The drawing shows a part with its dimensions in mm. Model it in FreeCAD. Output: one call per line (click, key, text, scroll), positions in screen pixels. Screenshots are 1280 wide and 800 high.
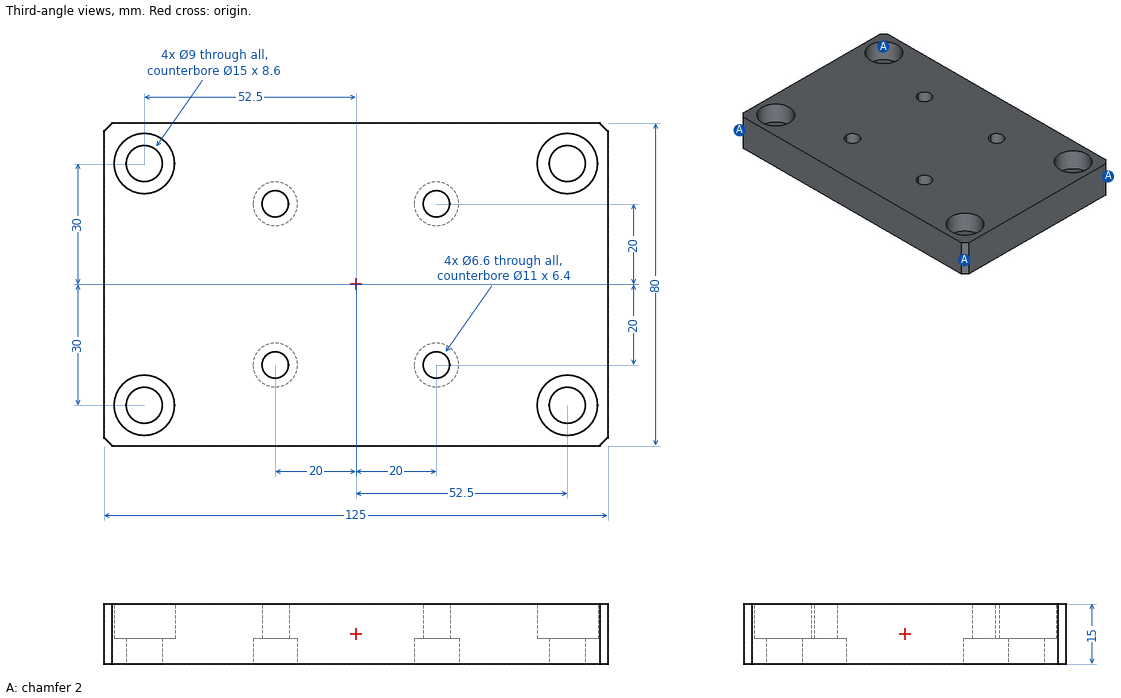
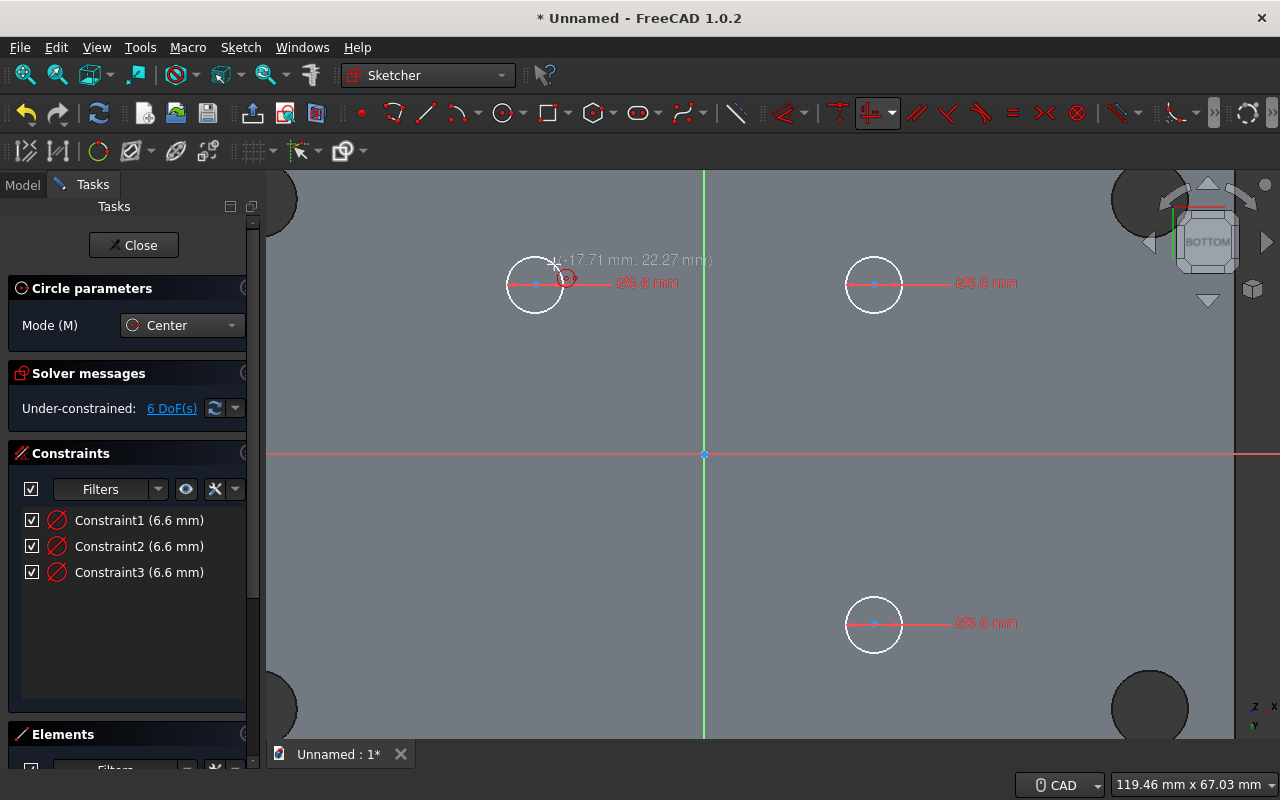
click(535, 624)
move(554, 604)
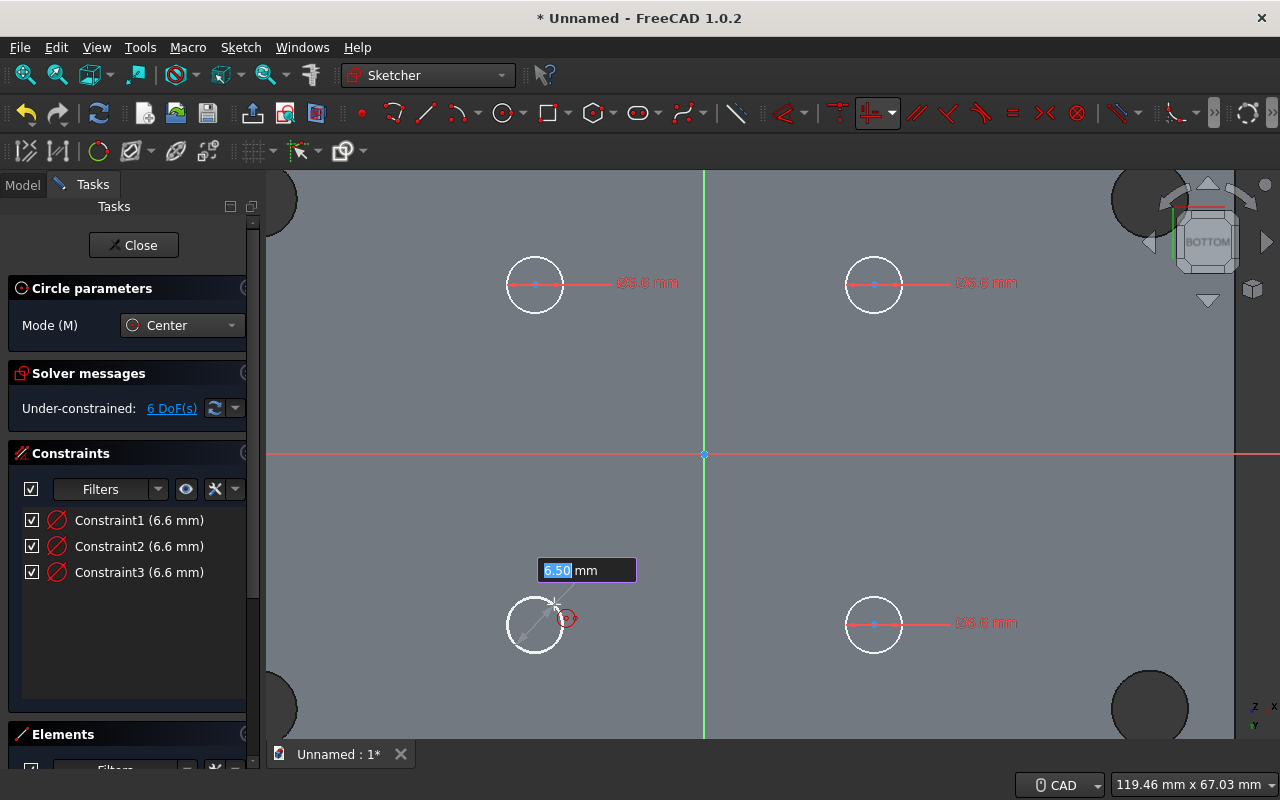
text(6.6)
key(Return)
key(Escape)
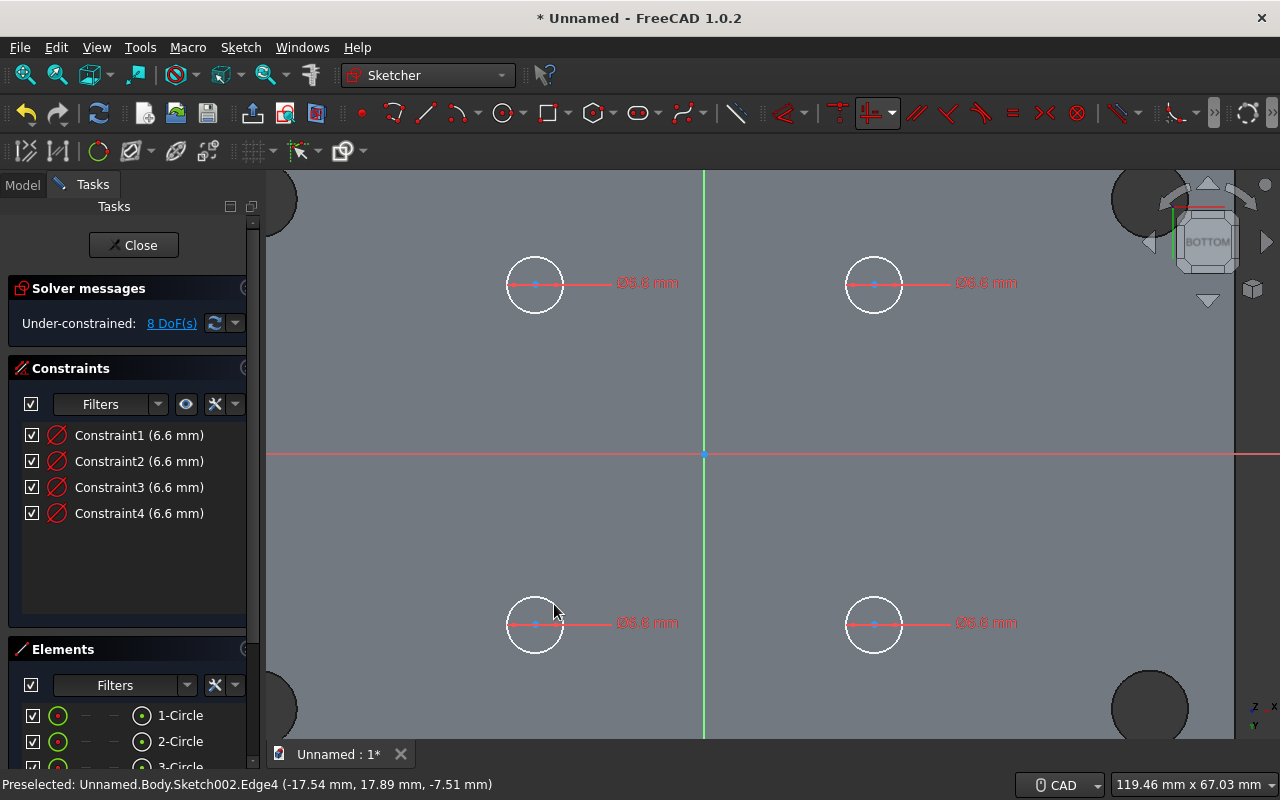
click(874, 285)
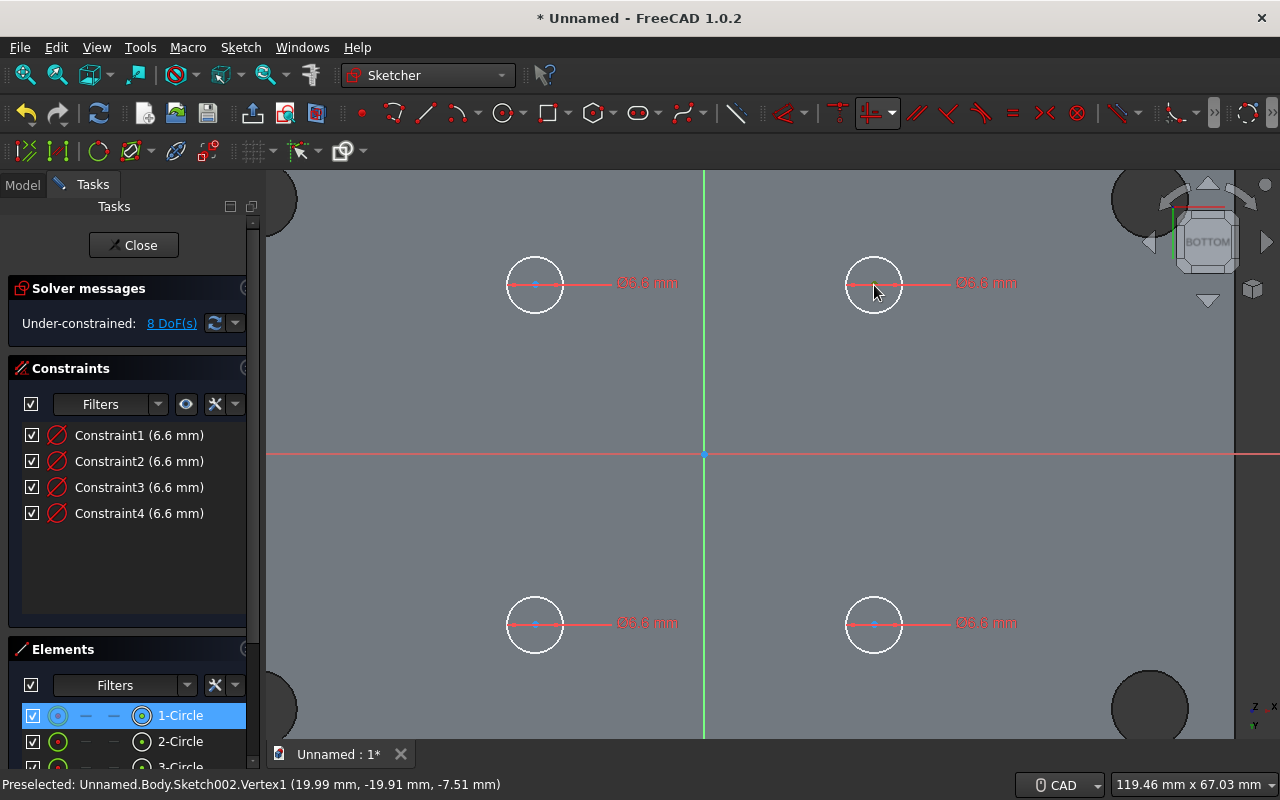
click(874, 625)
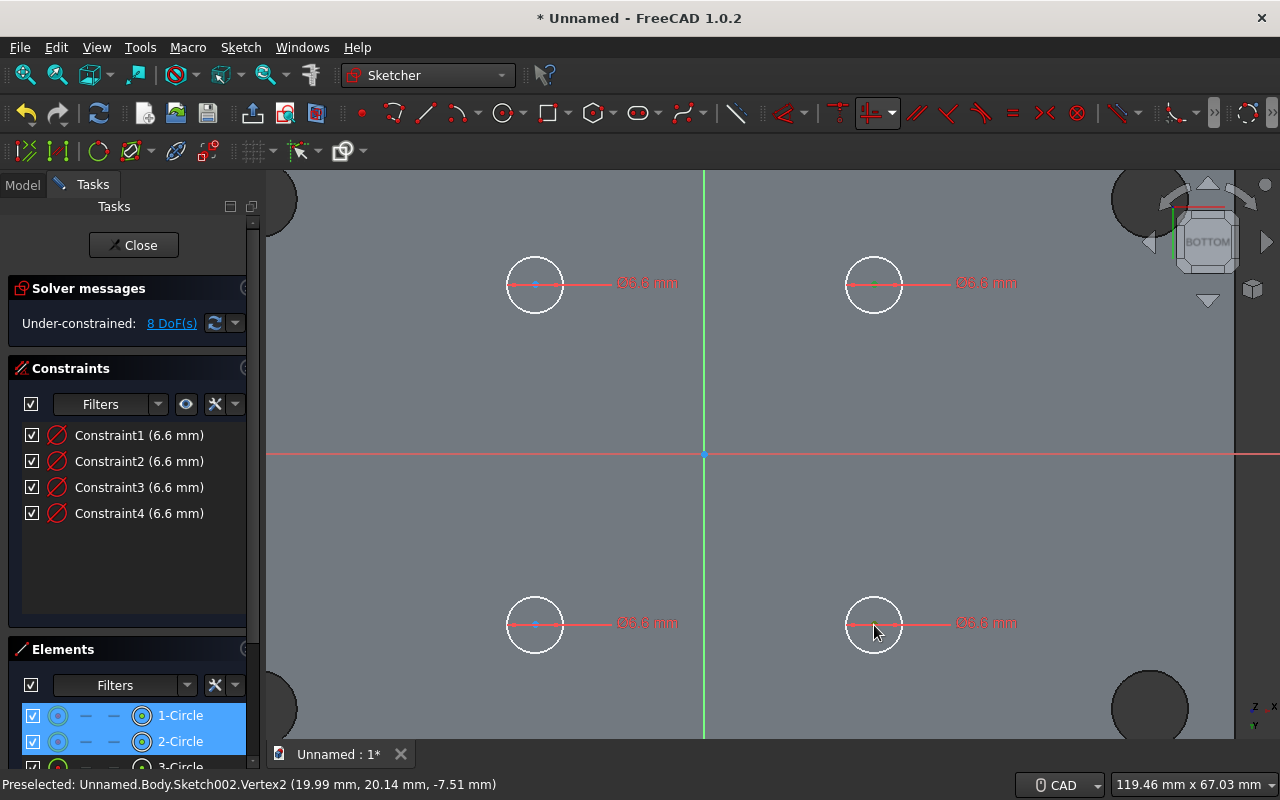
click(894, 114)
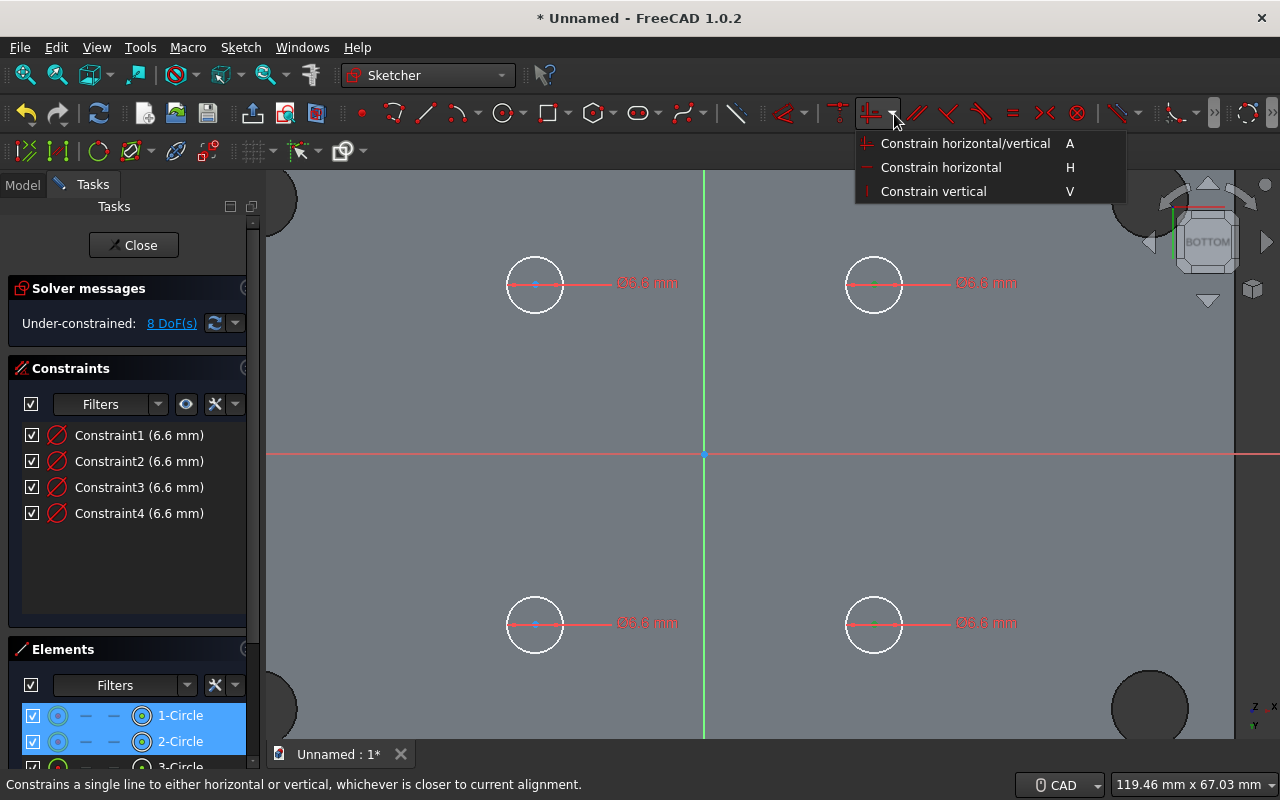
click(991, 191)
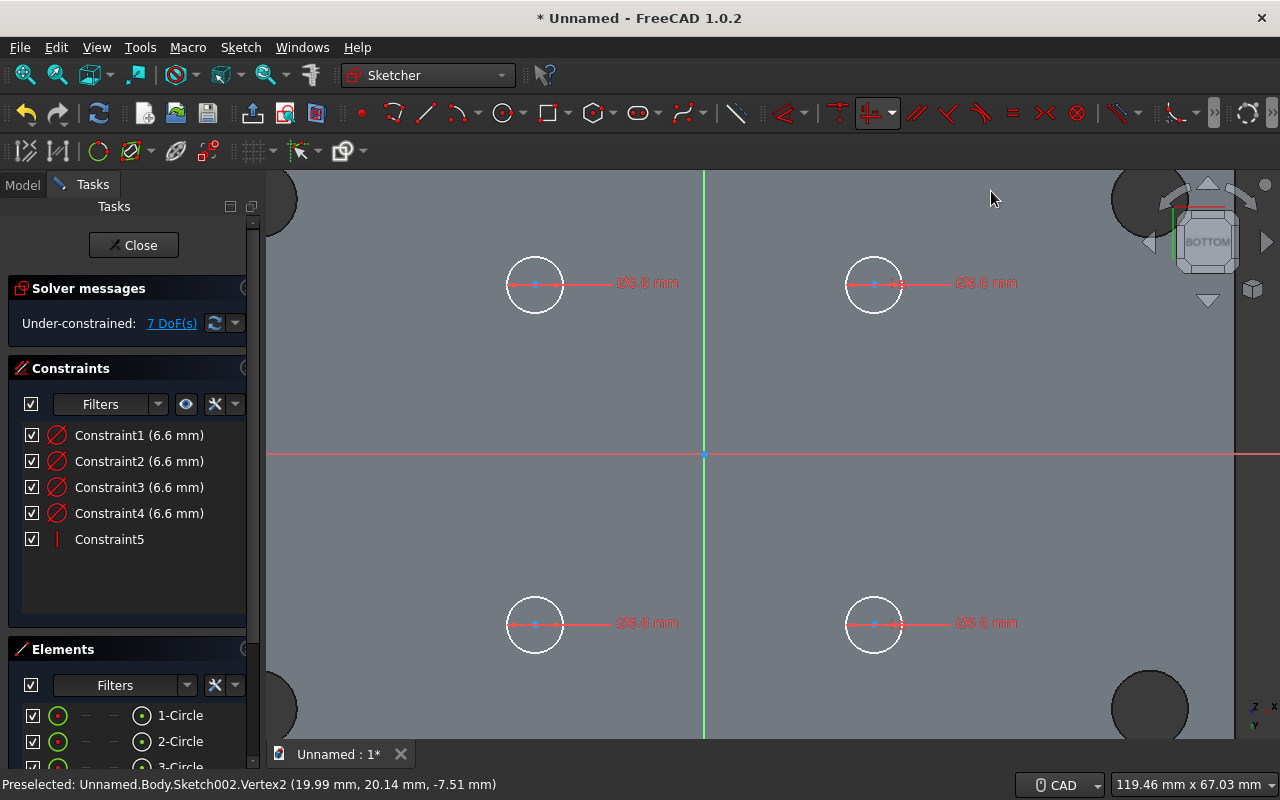
click(874, 285)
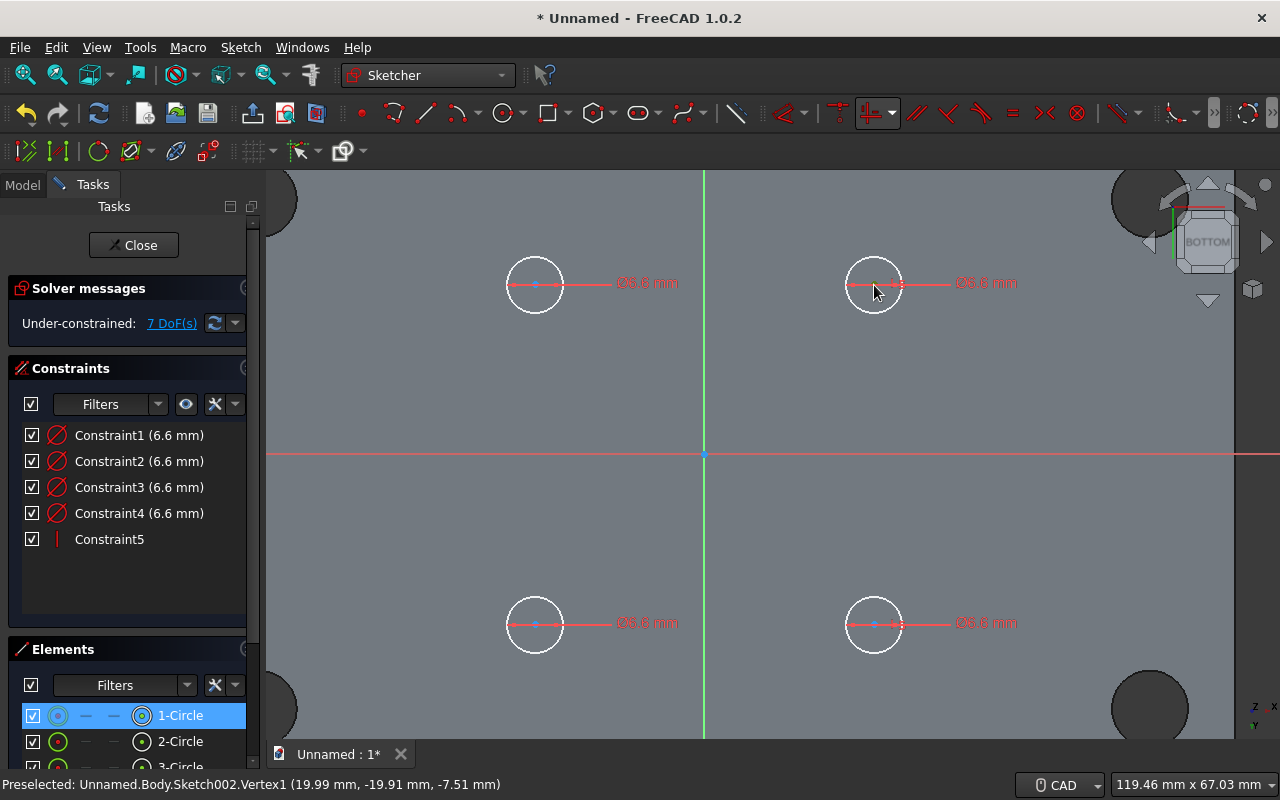
click(535, 285)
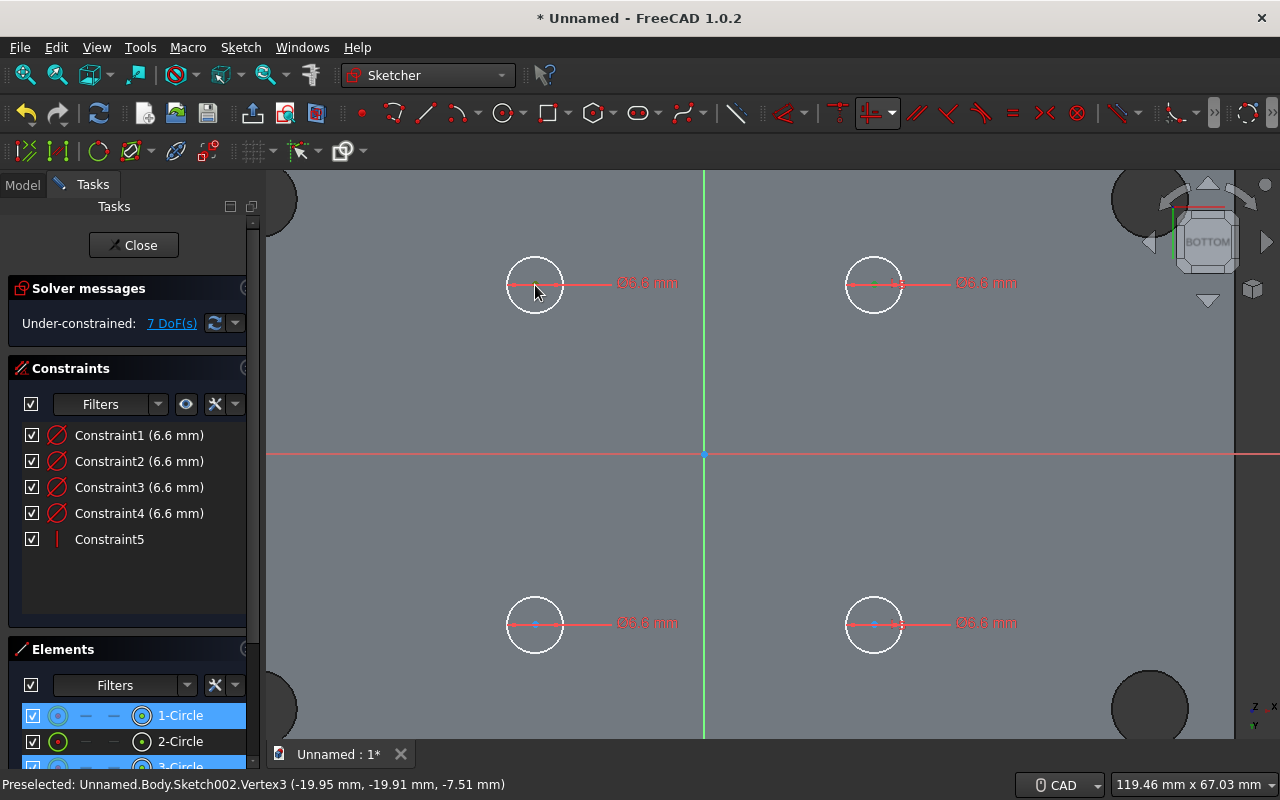
key(h)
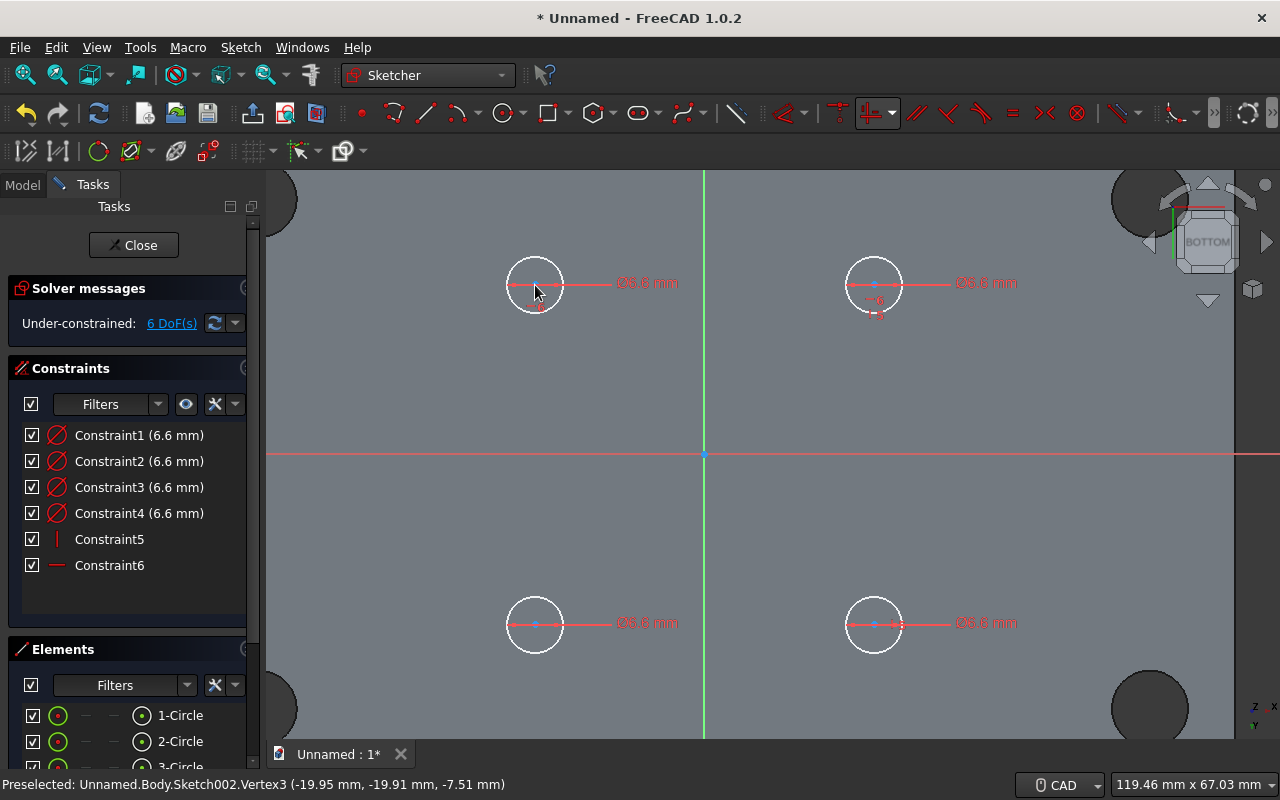
click(535, 285)